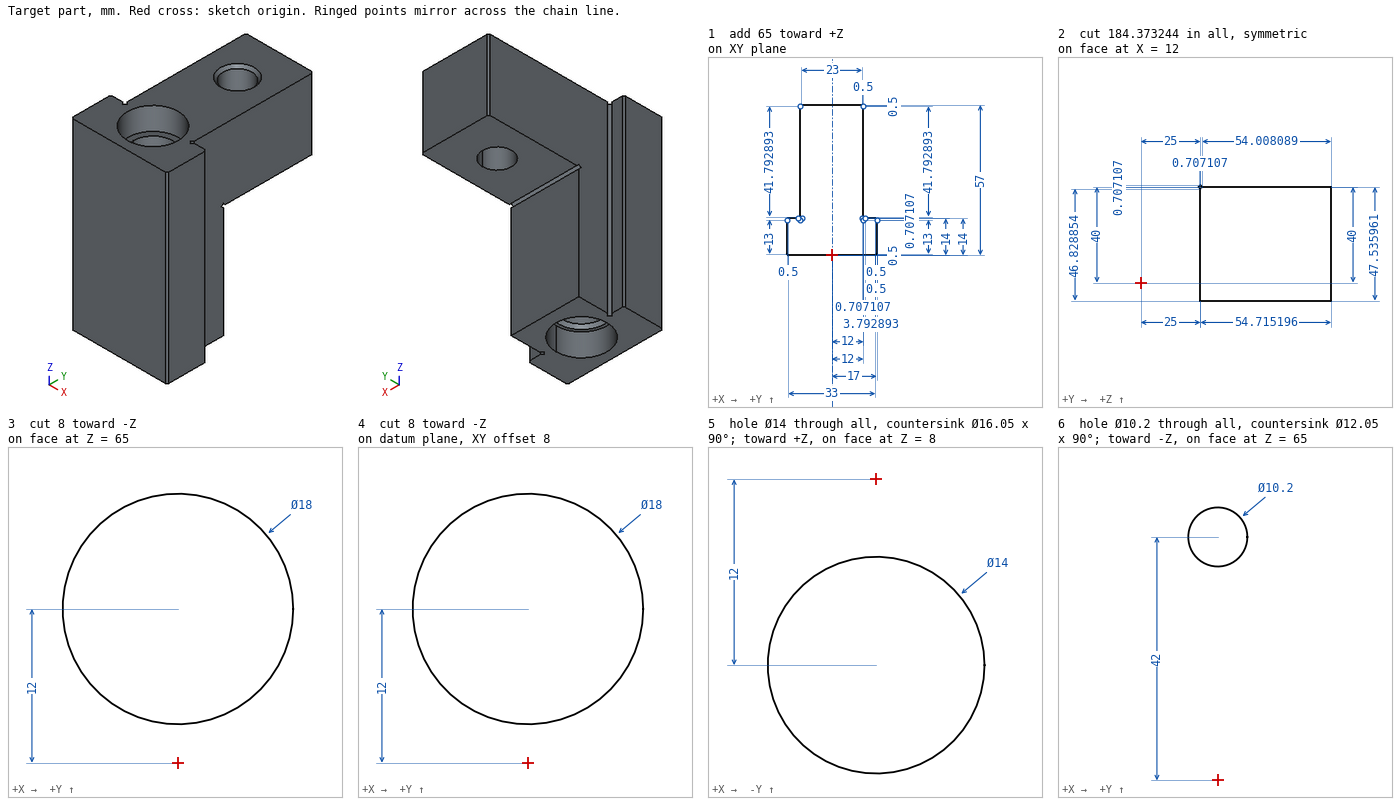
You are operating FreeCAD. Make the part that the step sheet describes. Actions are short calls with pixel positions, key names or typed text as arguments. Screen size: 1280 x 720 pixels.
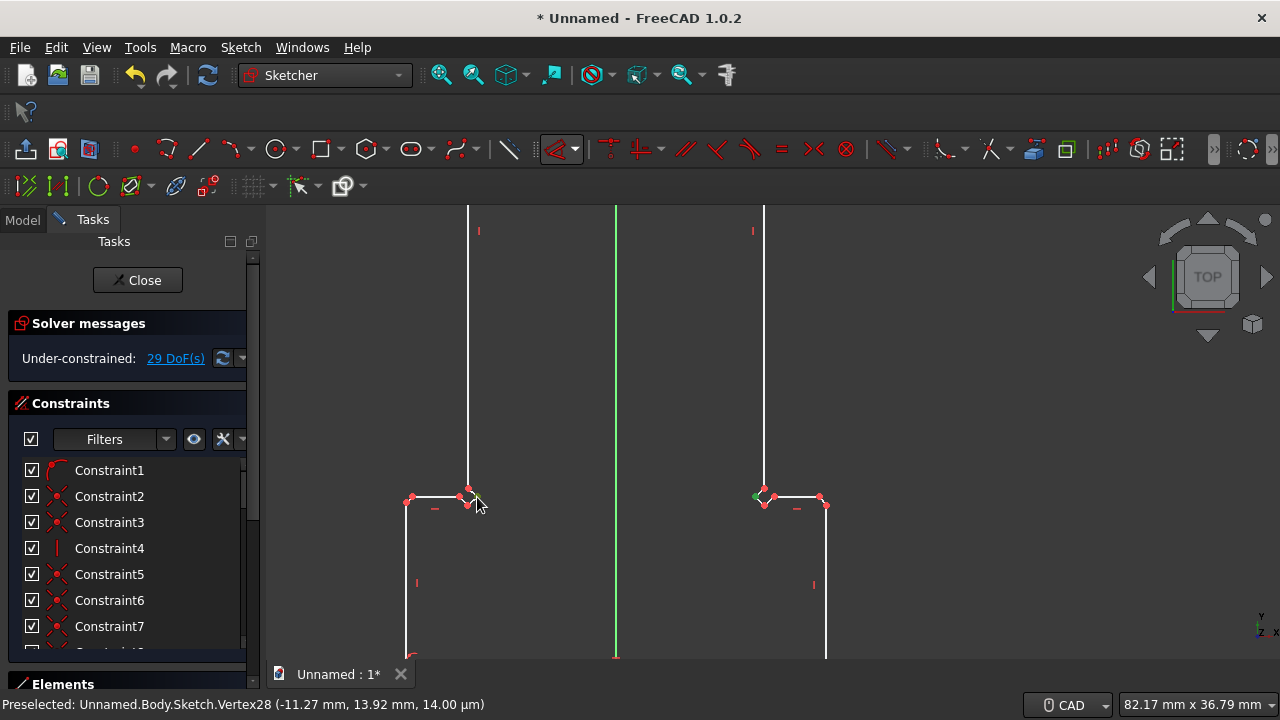
click(616, 603)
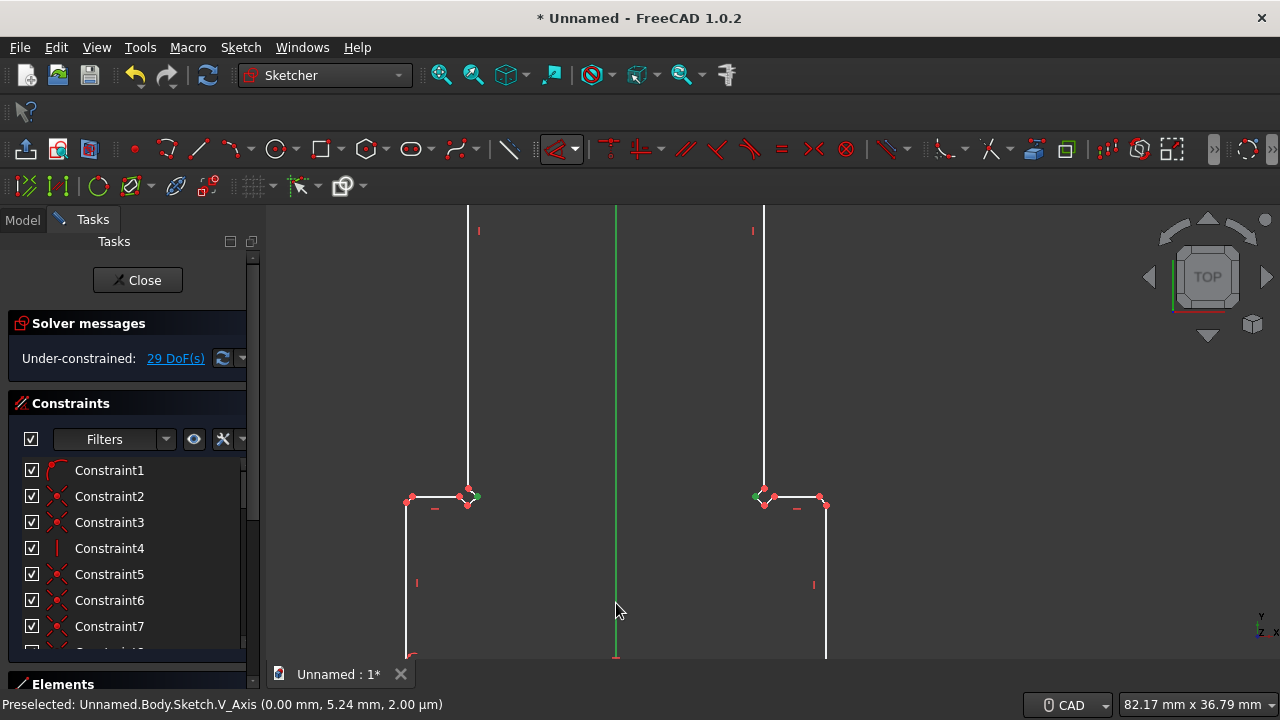
click(814, 150)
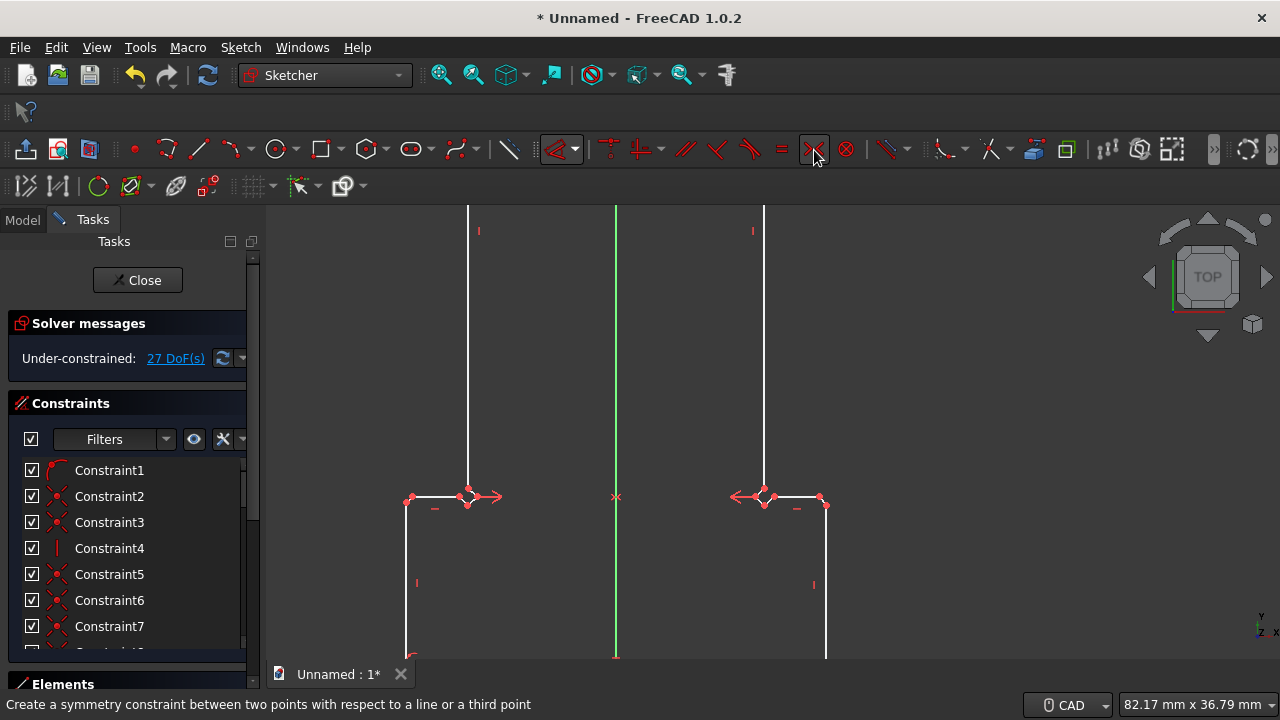
click(764, 506)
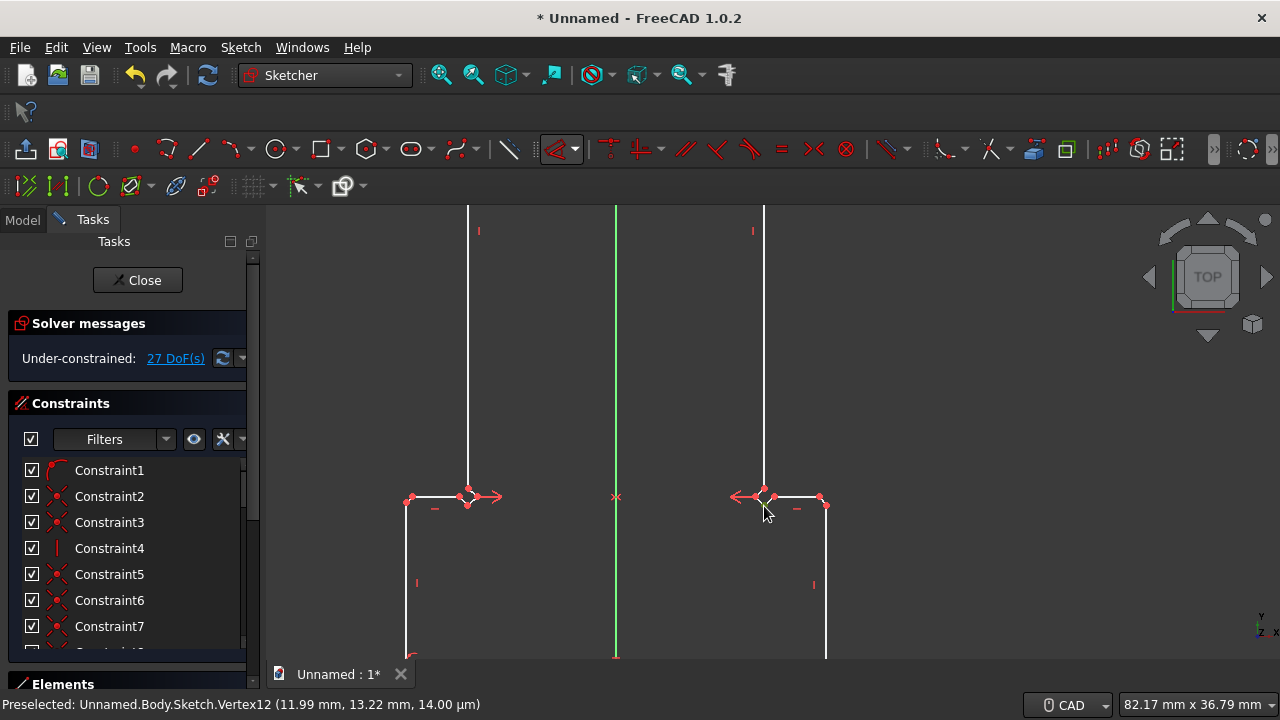
click(468, 506)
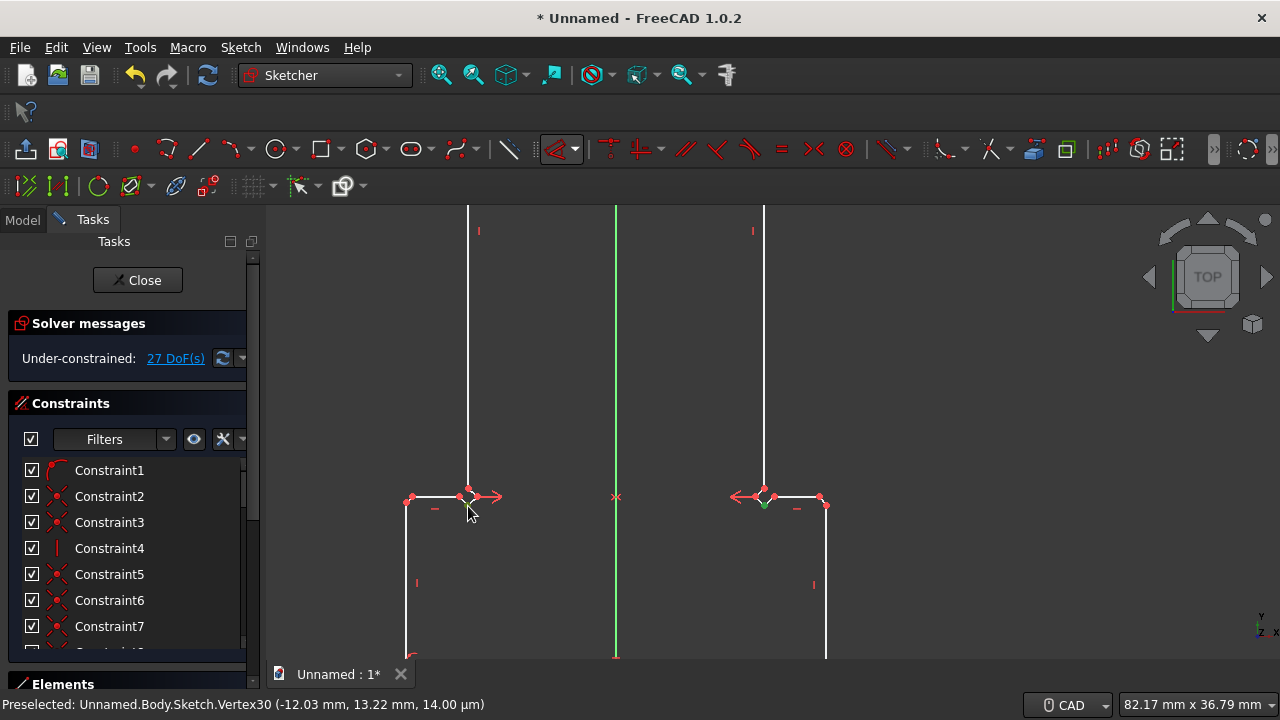
click(616, 603)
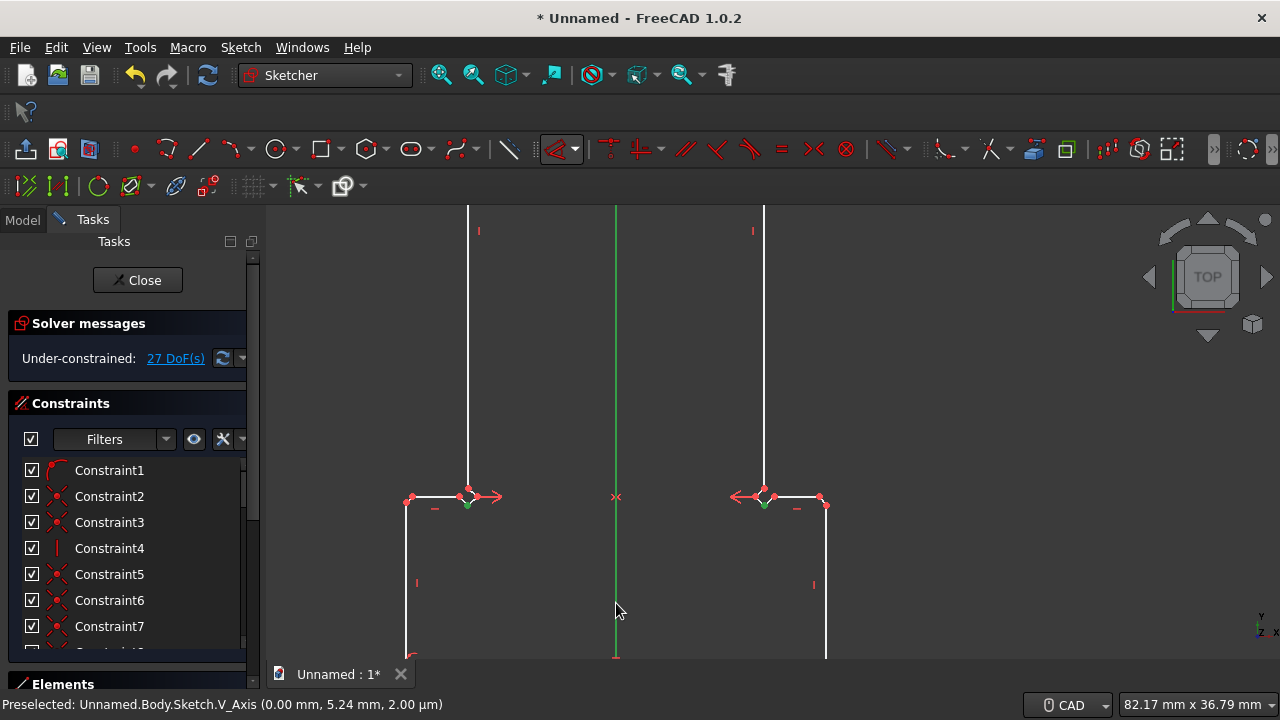
key(s)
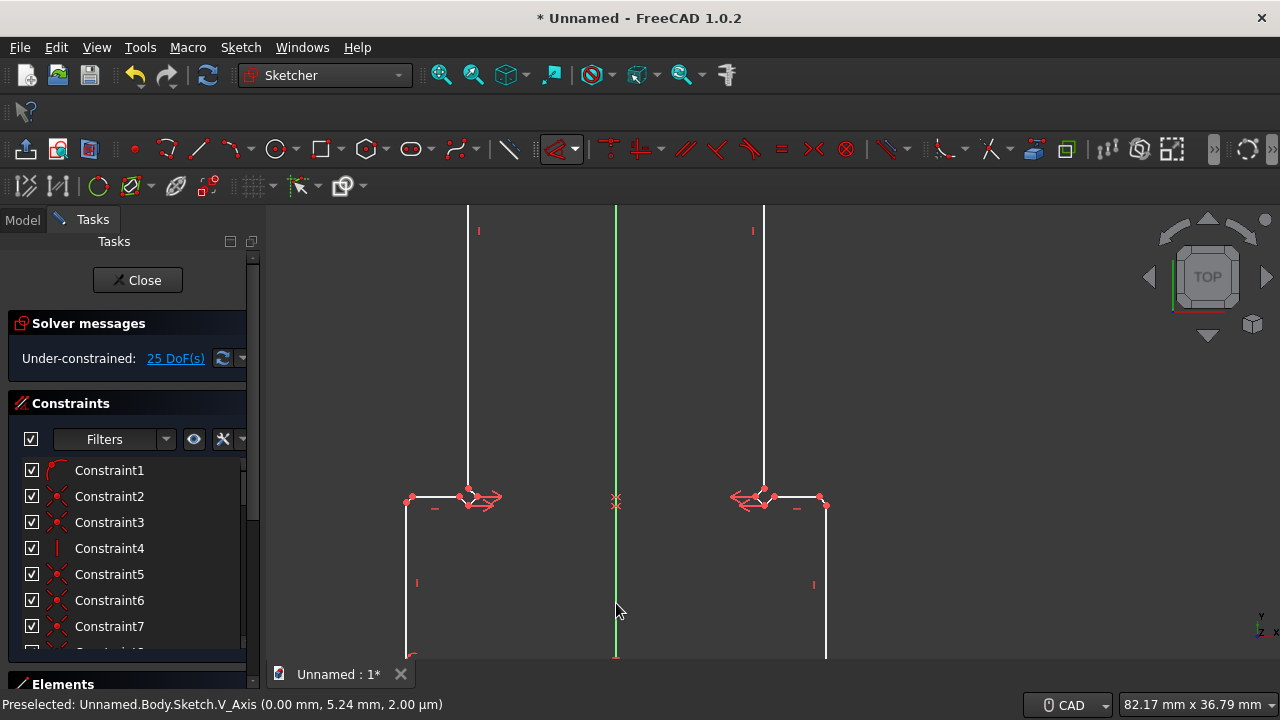
click(774, 497)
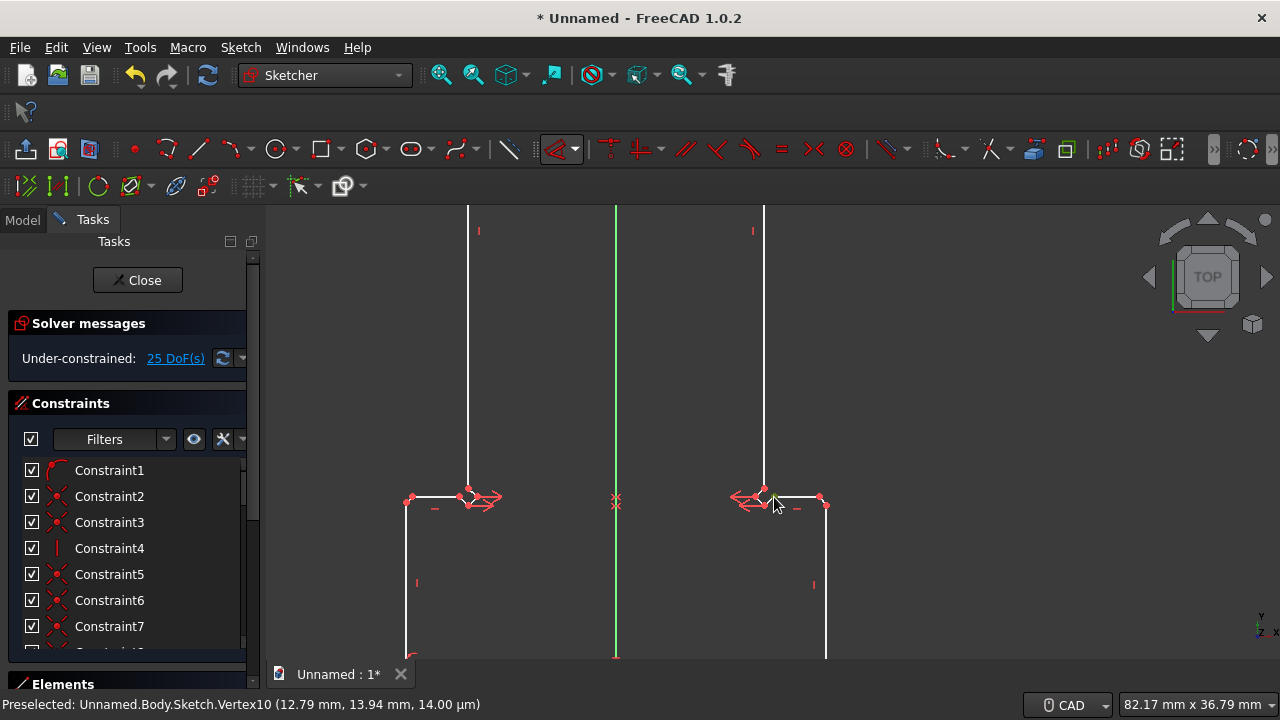
click(459, 497)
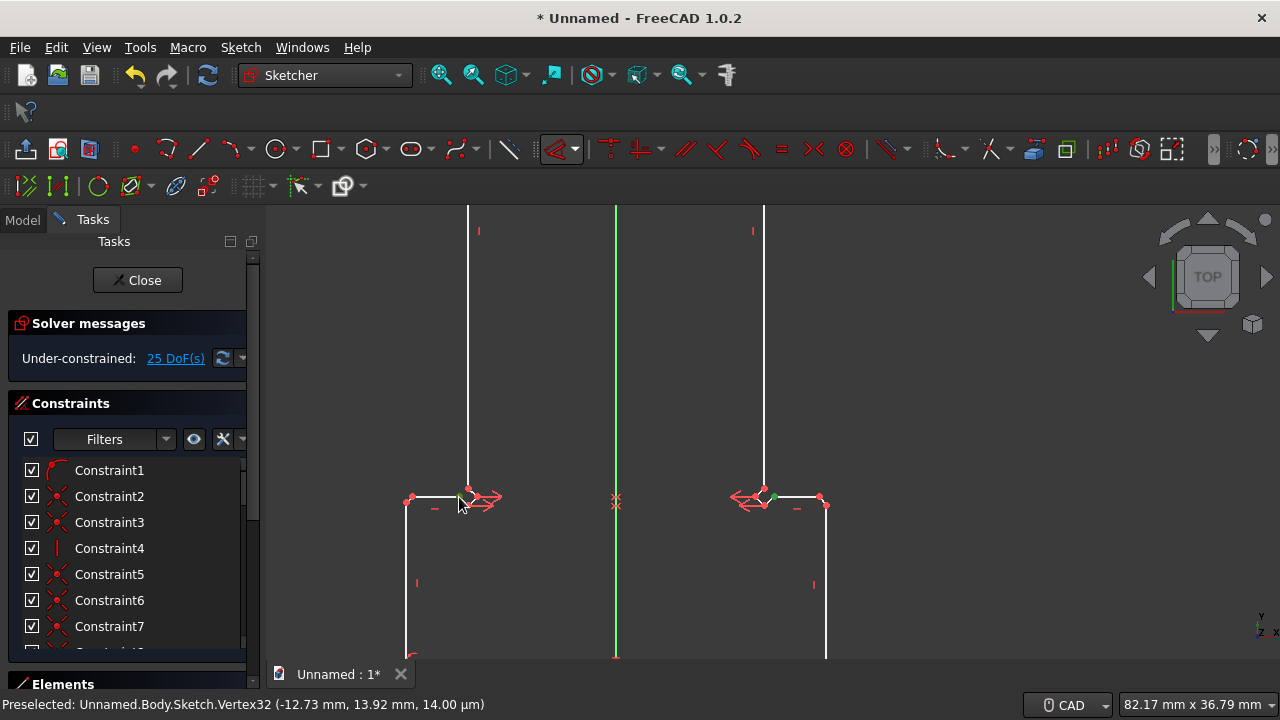
click(616, 603)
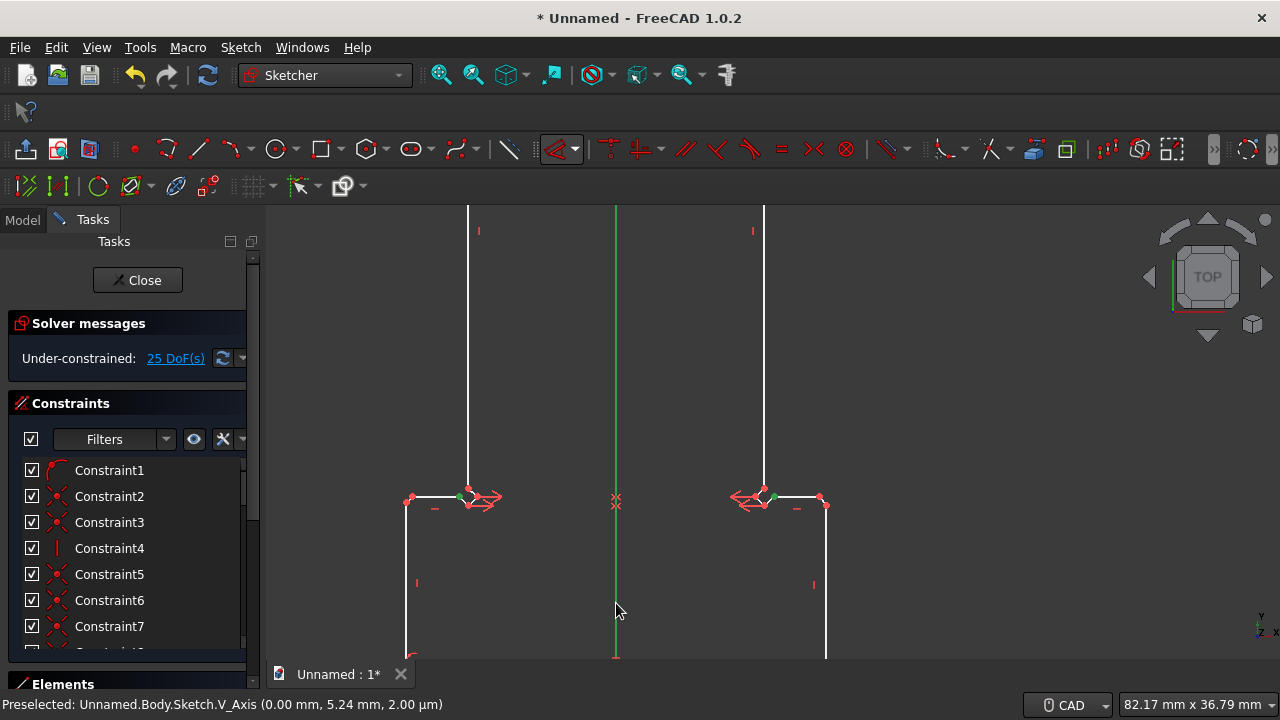
key(s)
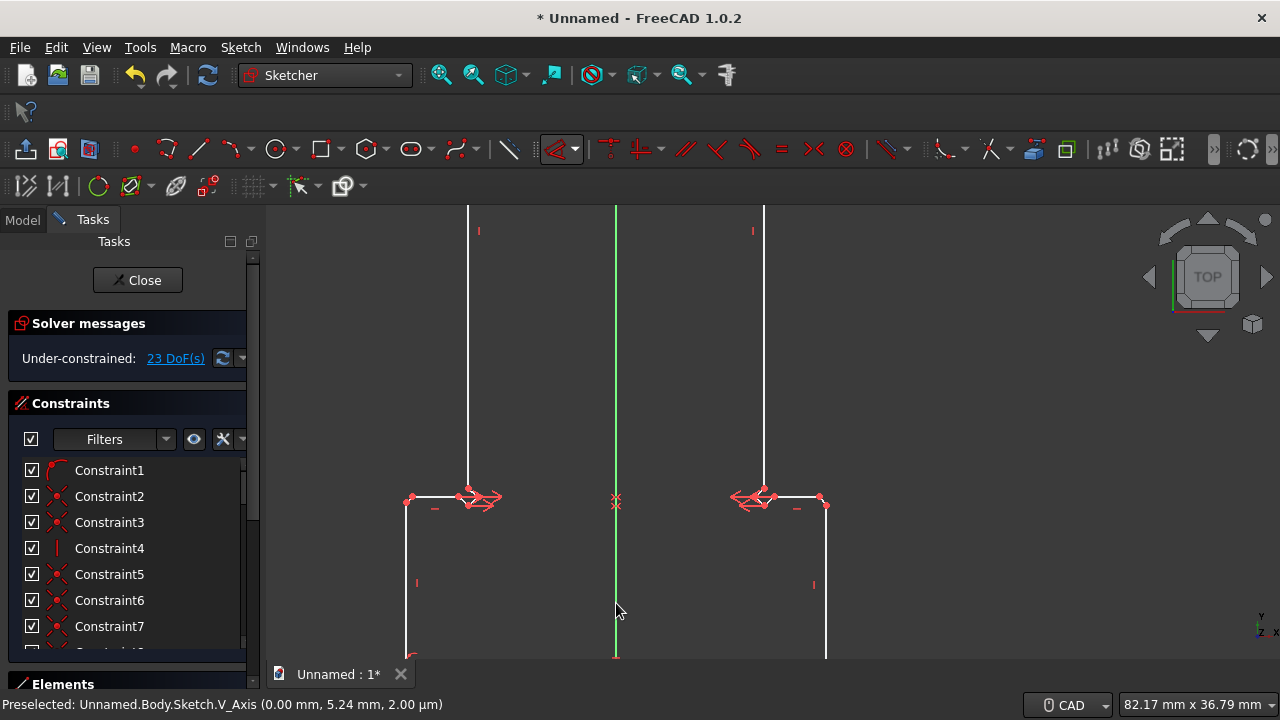
click(826, 506)